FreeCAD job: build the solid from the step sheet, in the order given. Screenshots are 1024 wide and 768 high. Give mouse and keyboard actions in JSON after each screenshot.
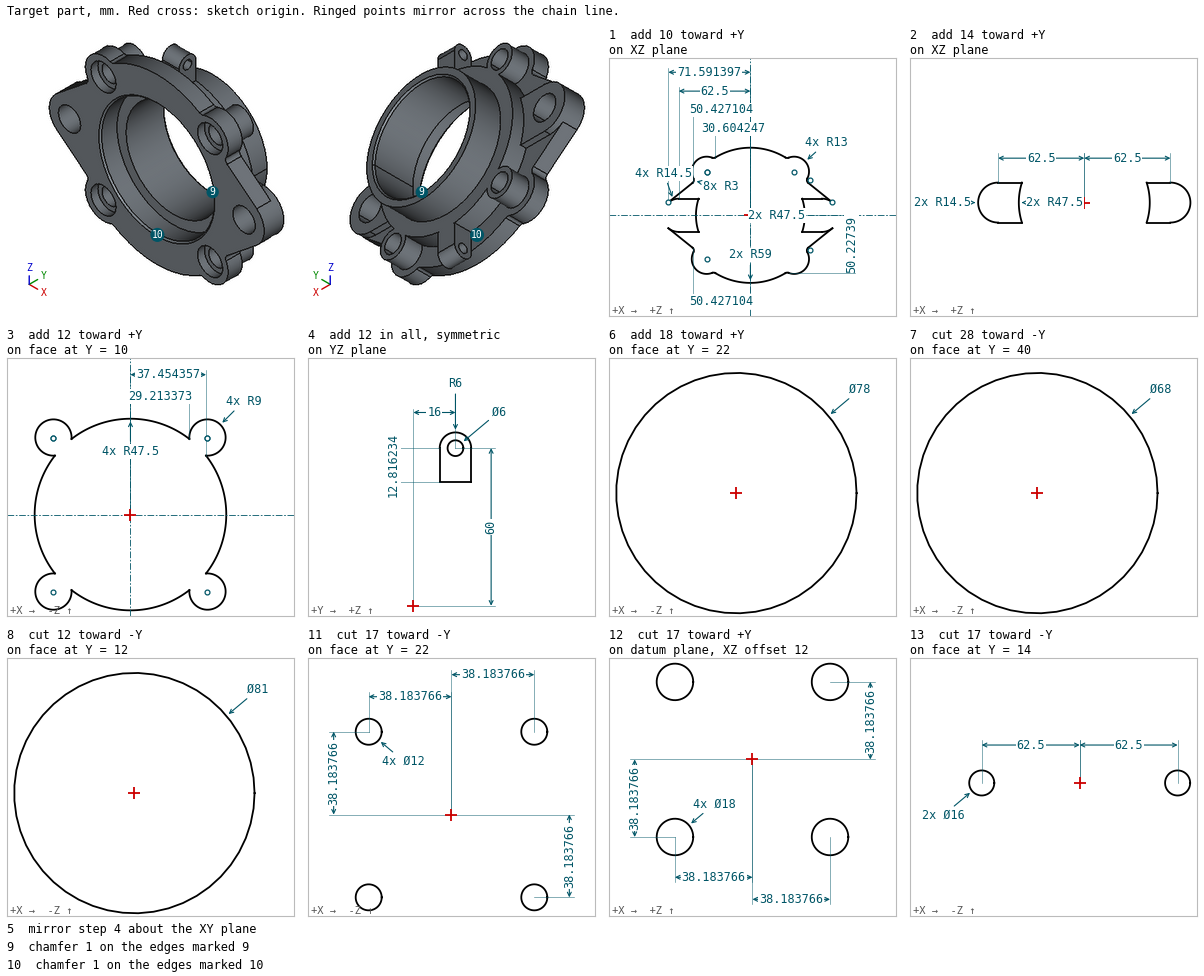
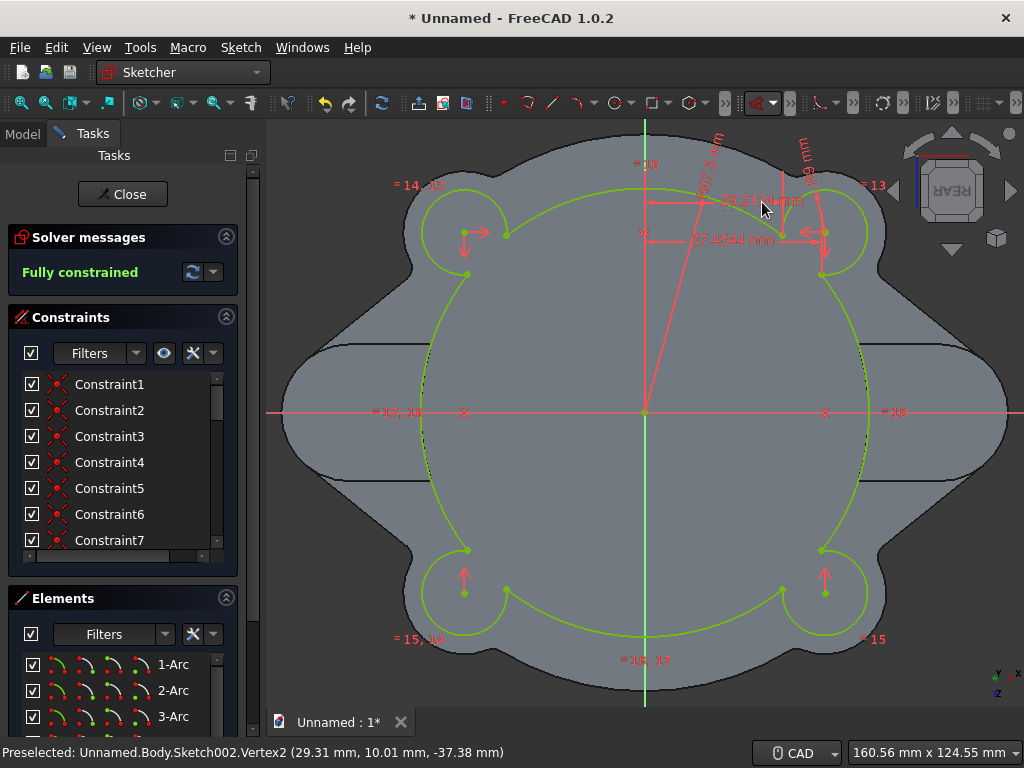
{"action": "left_click", "coordinate": [123, 194]}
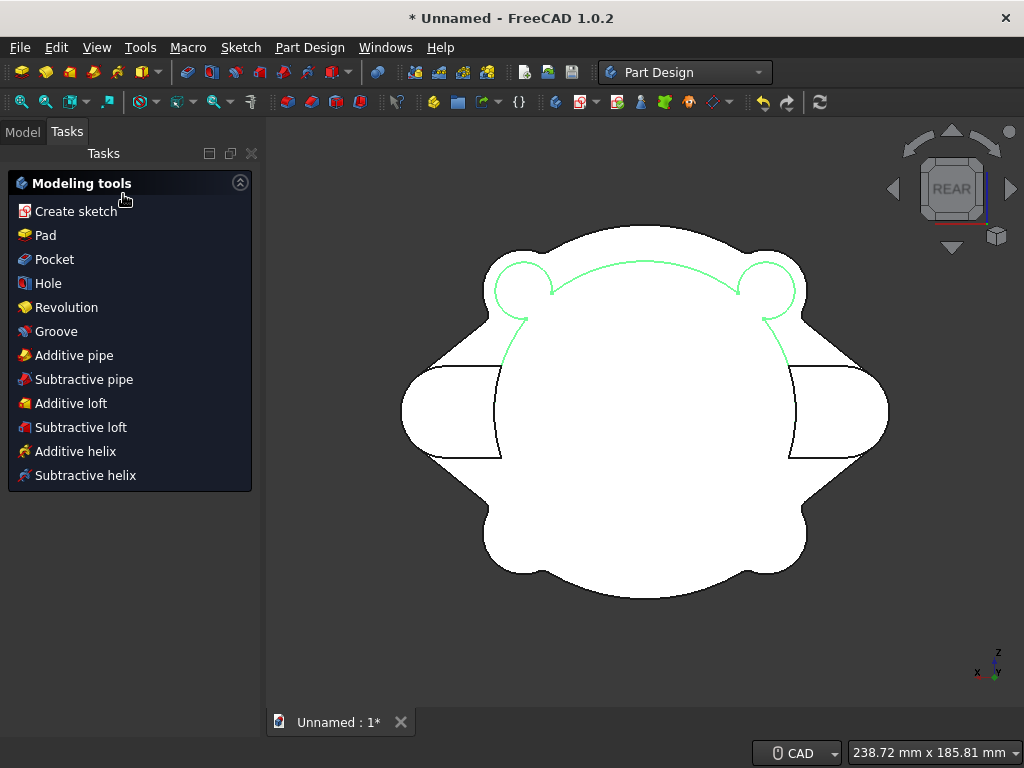
{"action": "left_click", "coordinate": [22, 72]}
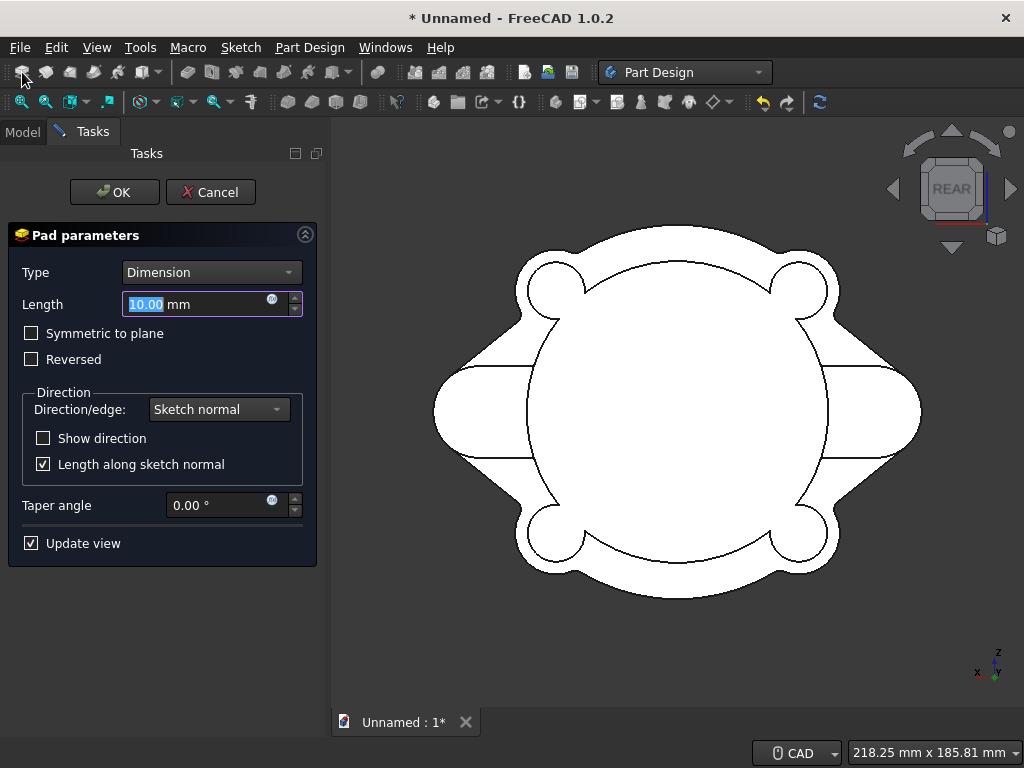
{"action": "type", "text": "12"}
{"action": "key", "text": "Tab"}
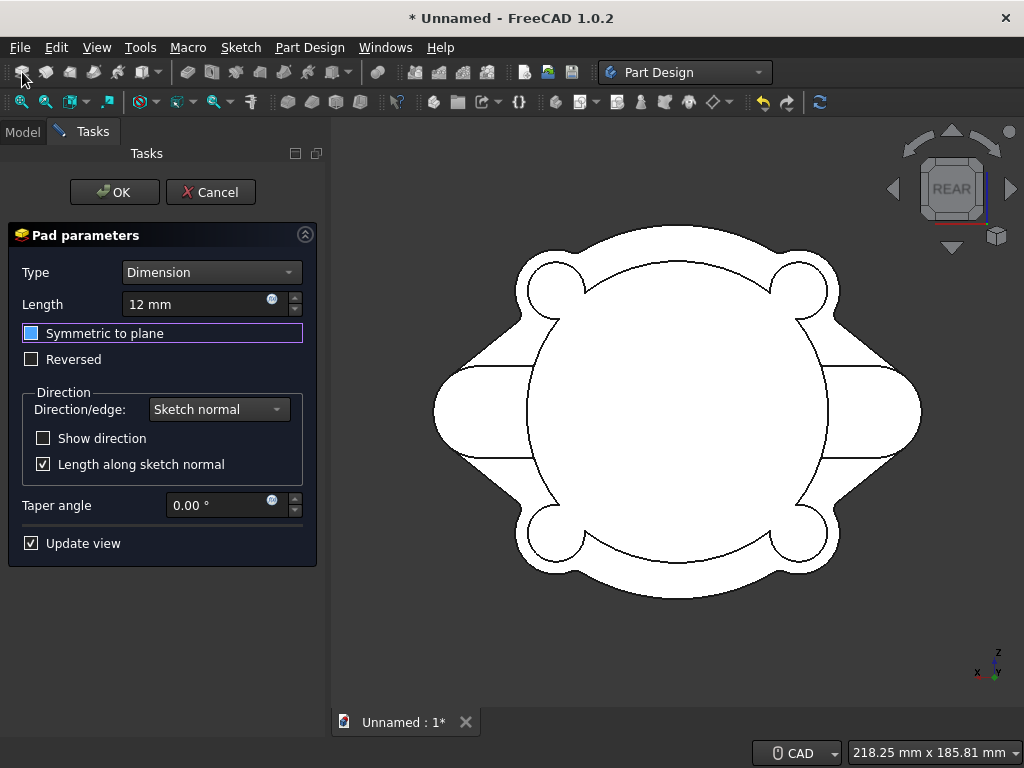
{"action": "left_click", "coordinate": [115, 192]}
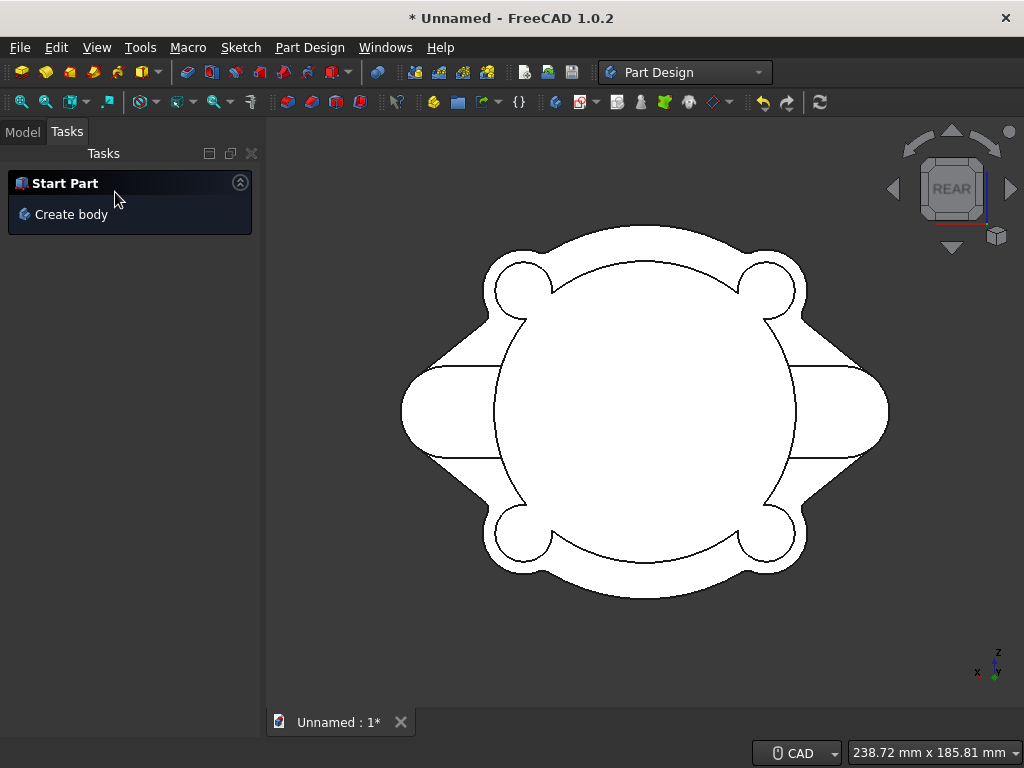
{"action": "left_click", "coordinate": [580, 102]}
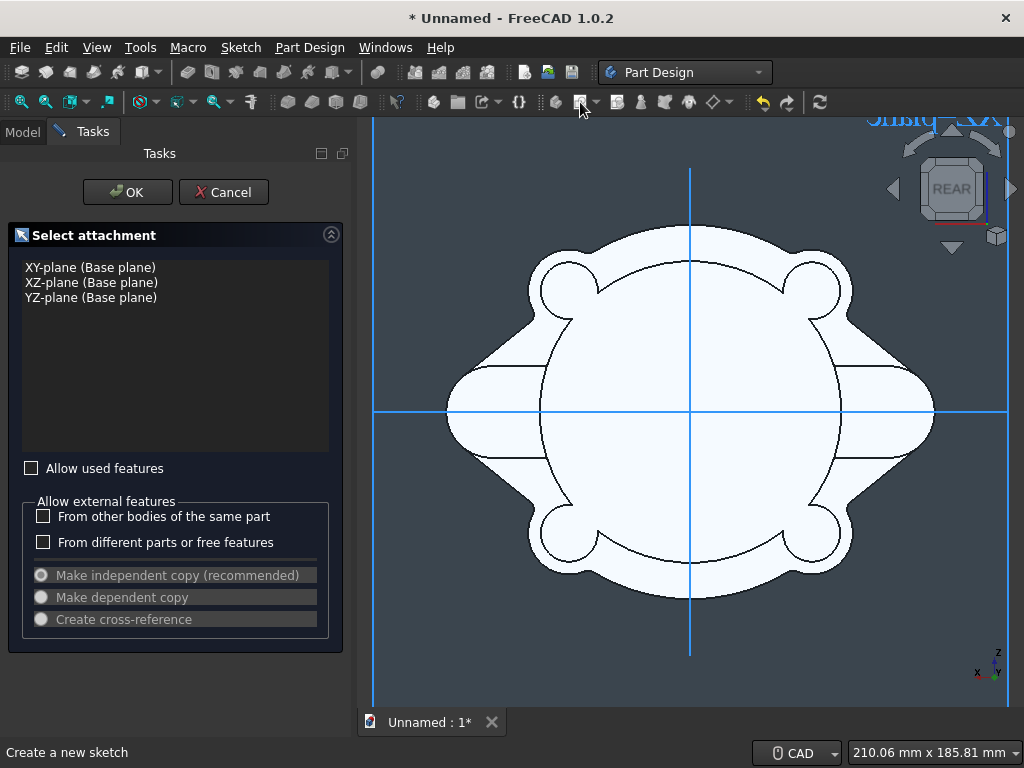
{"action": "left_click", "coordinate": [82, 298]}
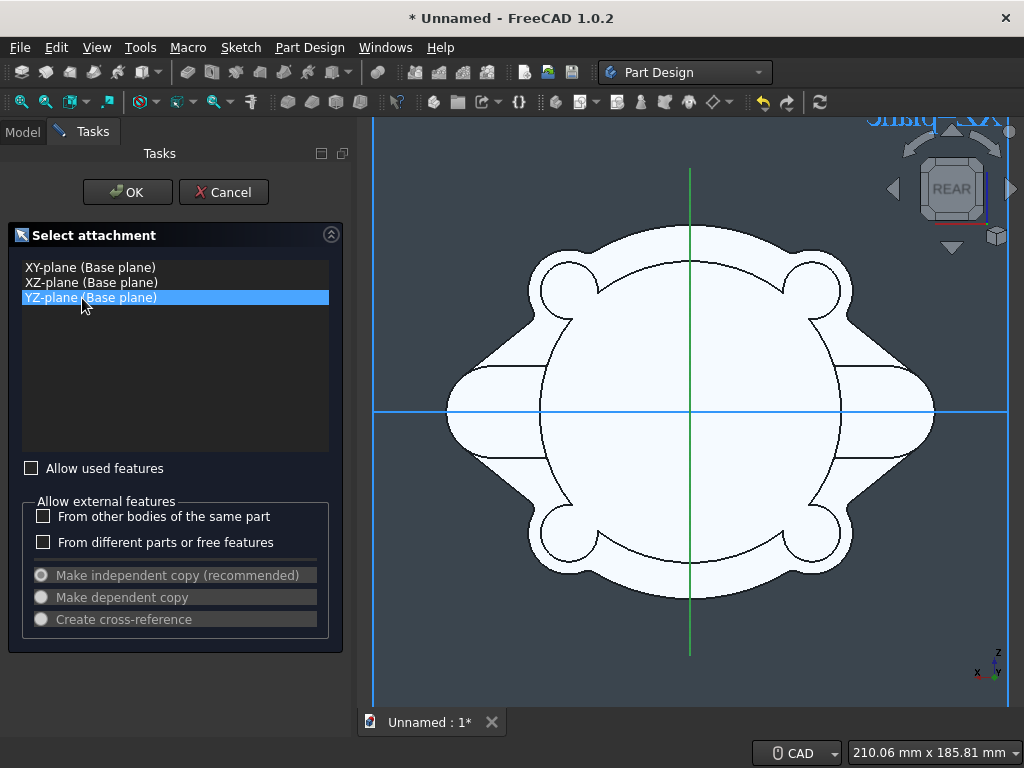
{"action": "left_click", "coordinate": [128, 192]}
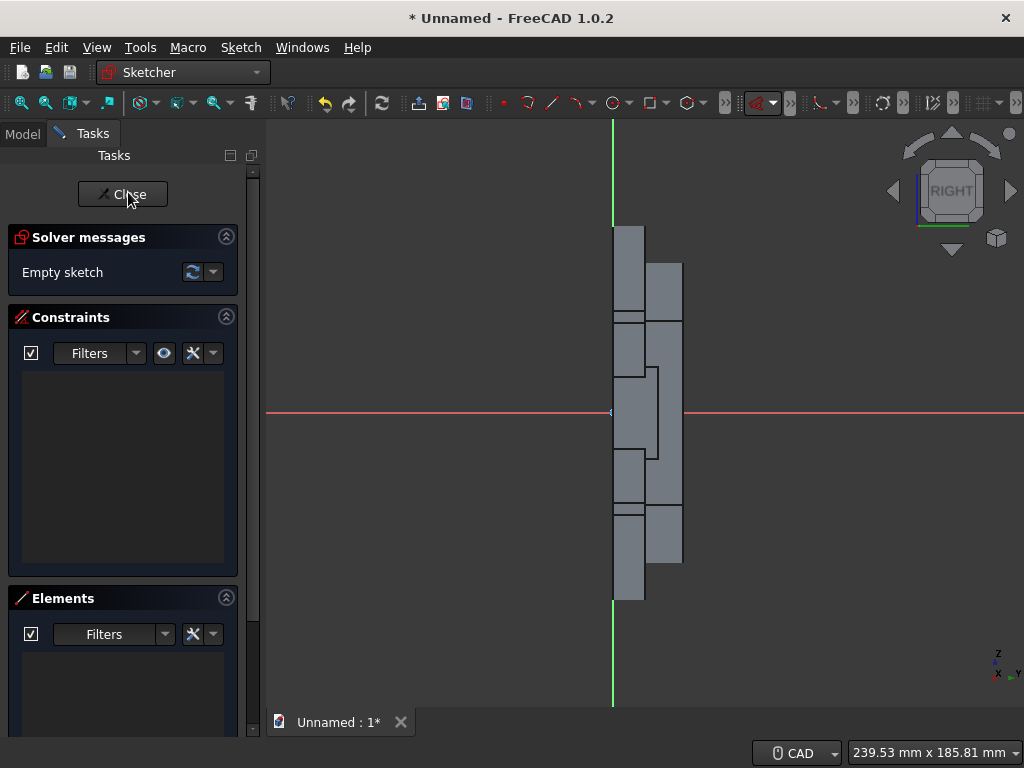
{"action": "key", "text": "q s"}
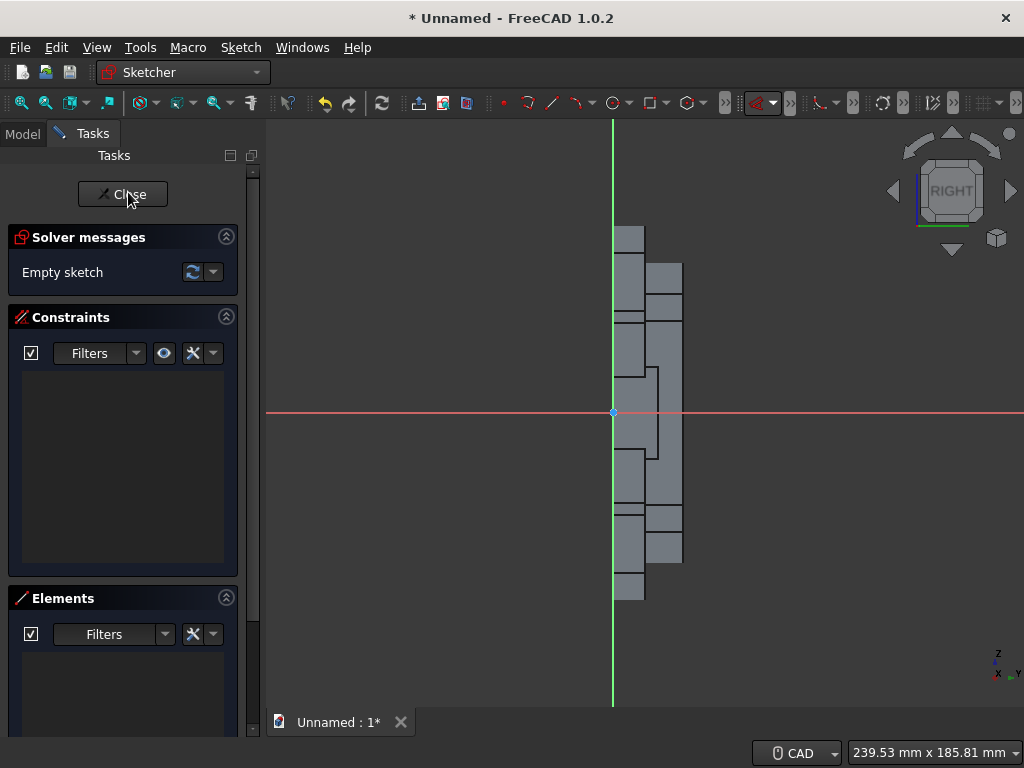
{"action": "scroll", "coordinate": [681, 198], "scroll_direction": "up", "scroll_amount": 9}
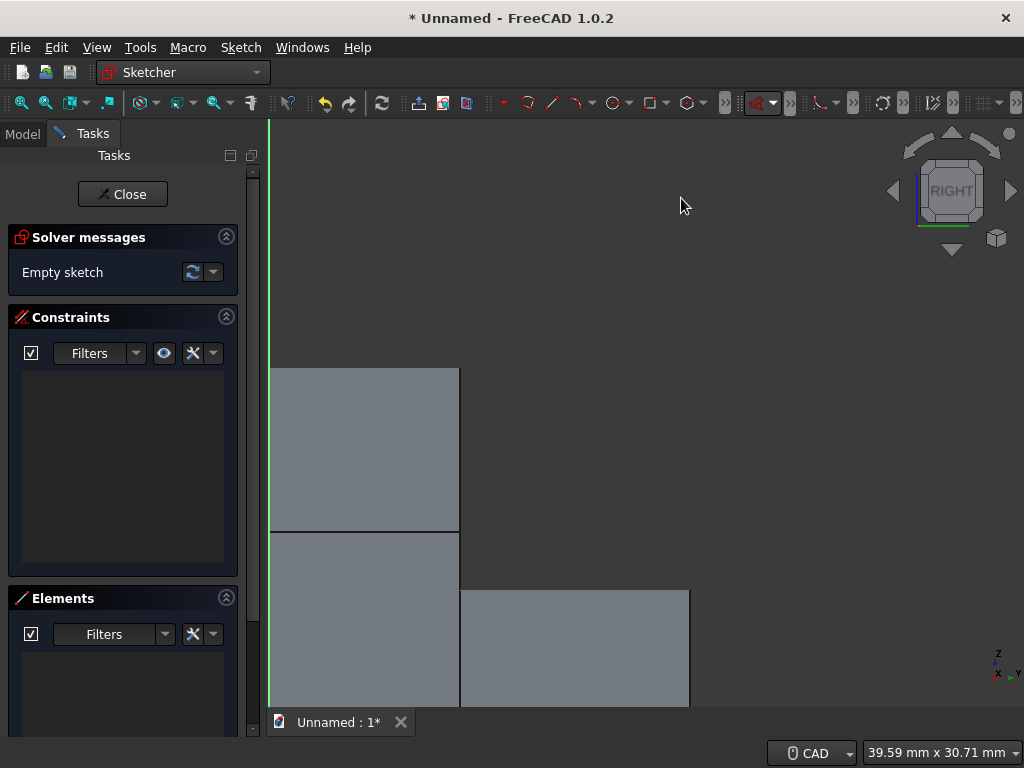
{"action": "key", "text": "g m"}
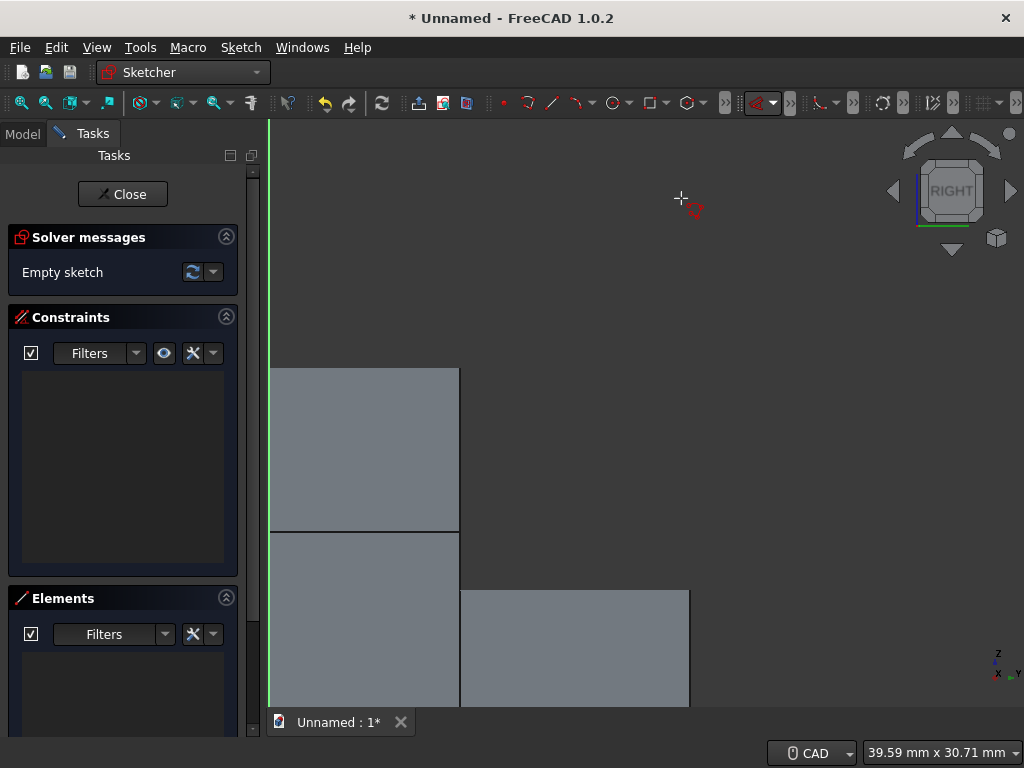
{"action": "left_click", "coordinate": [460, 349]}
{"action": "left_click", "coordinate": [460, 595]}
{"action": "left_click", "coordinate": [690, 595]}
{"action": "left_click", "coordinate": [690, 349]}
{"action": "right_click", "coordinate": [690, 349]}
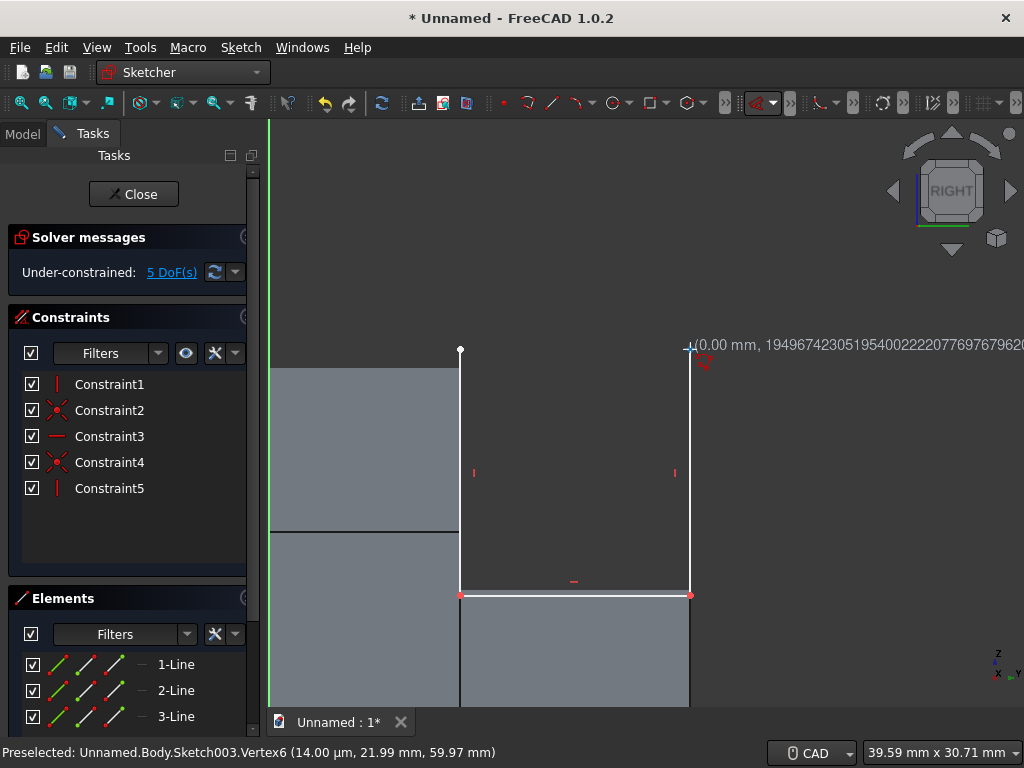
{"action": "key", "text": "g 3 a"}